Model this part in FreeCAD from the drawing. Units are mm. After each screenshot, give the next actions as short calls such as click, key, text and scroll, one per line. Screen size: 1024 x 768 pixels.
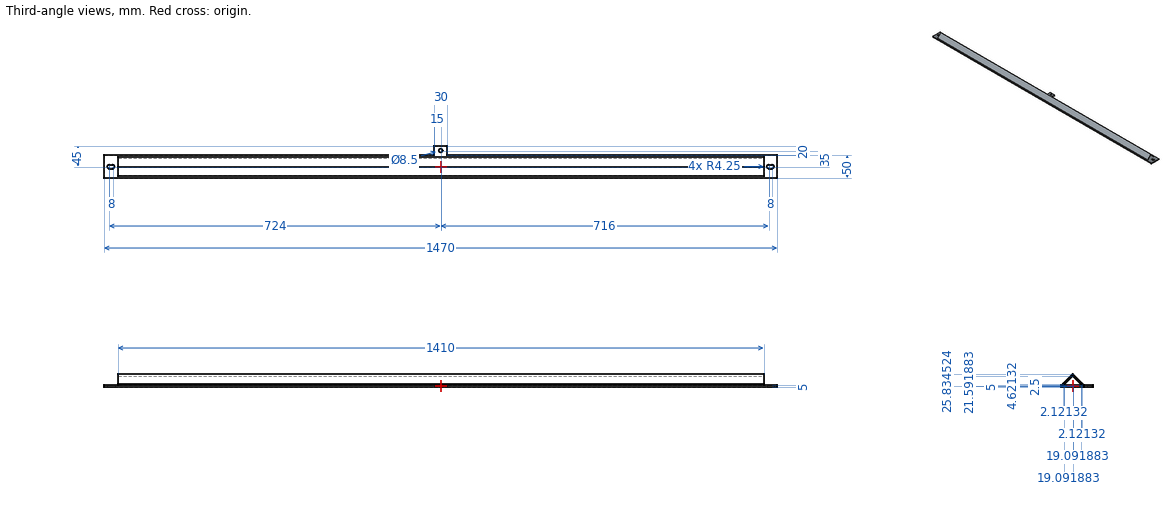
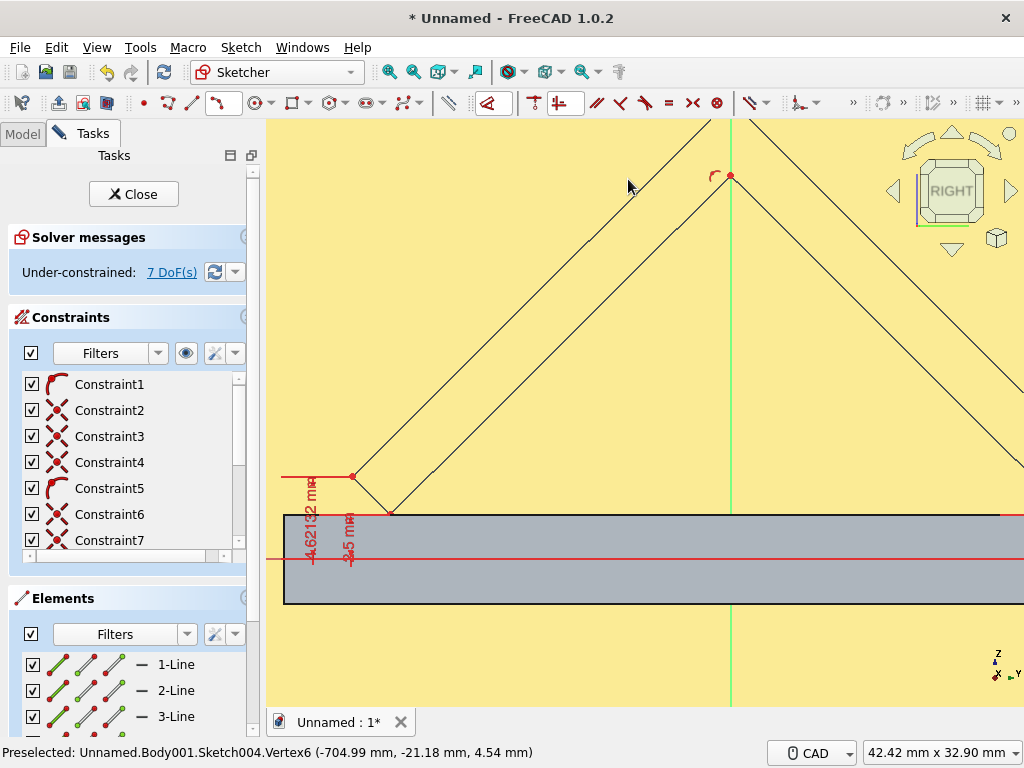
scroll(389, 516, down, 3)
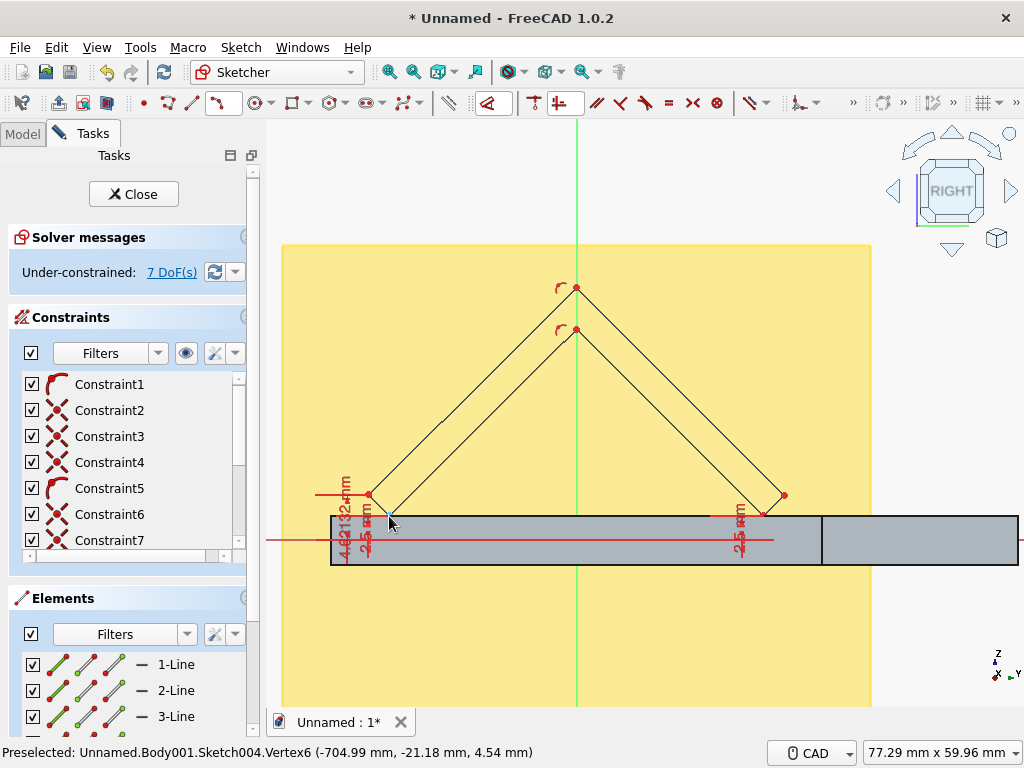
click(784, 496)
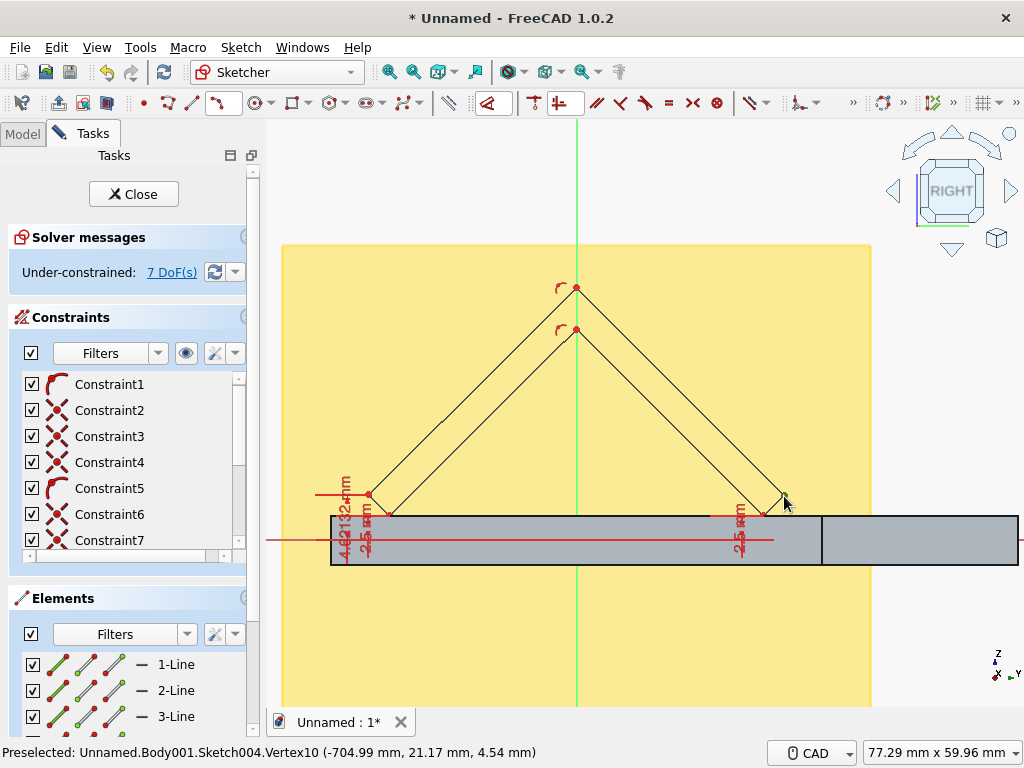
key(i)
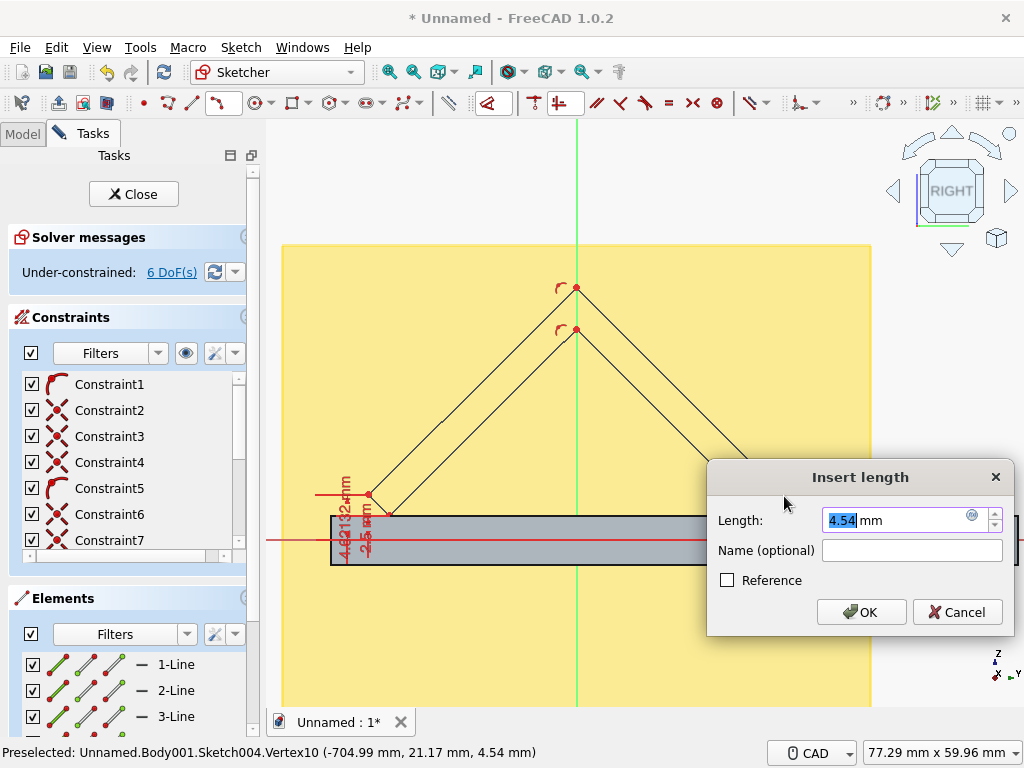
text(4.62132)
key(Return)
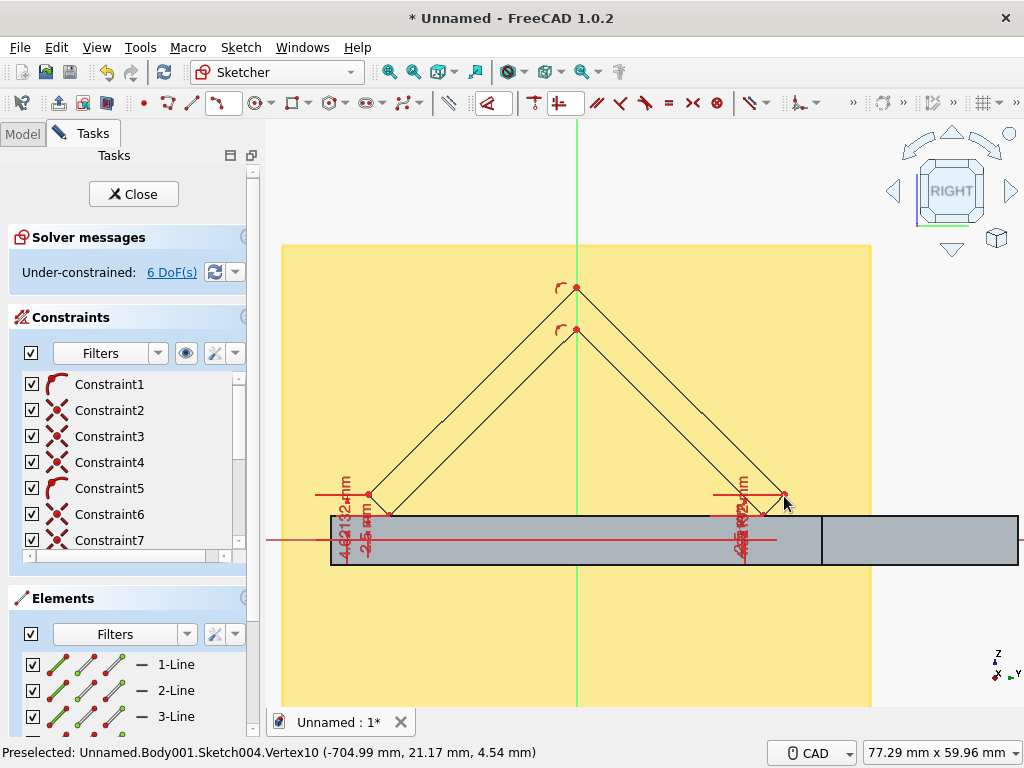
scroll(381, 507, up, 4)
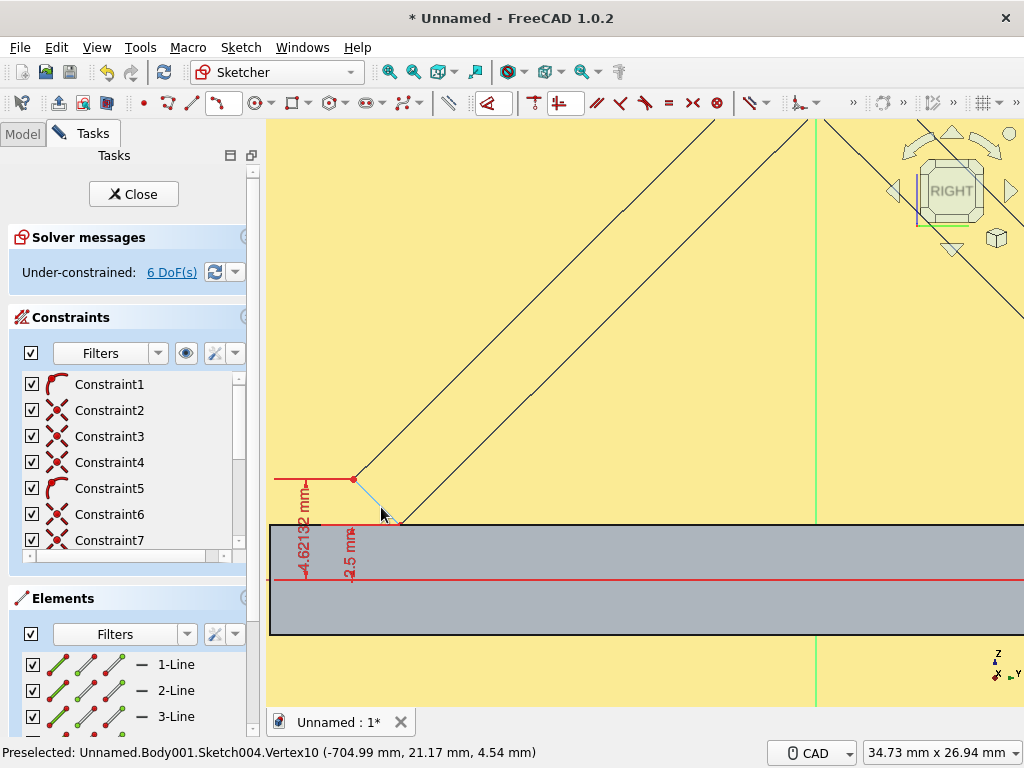
click(382, 507)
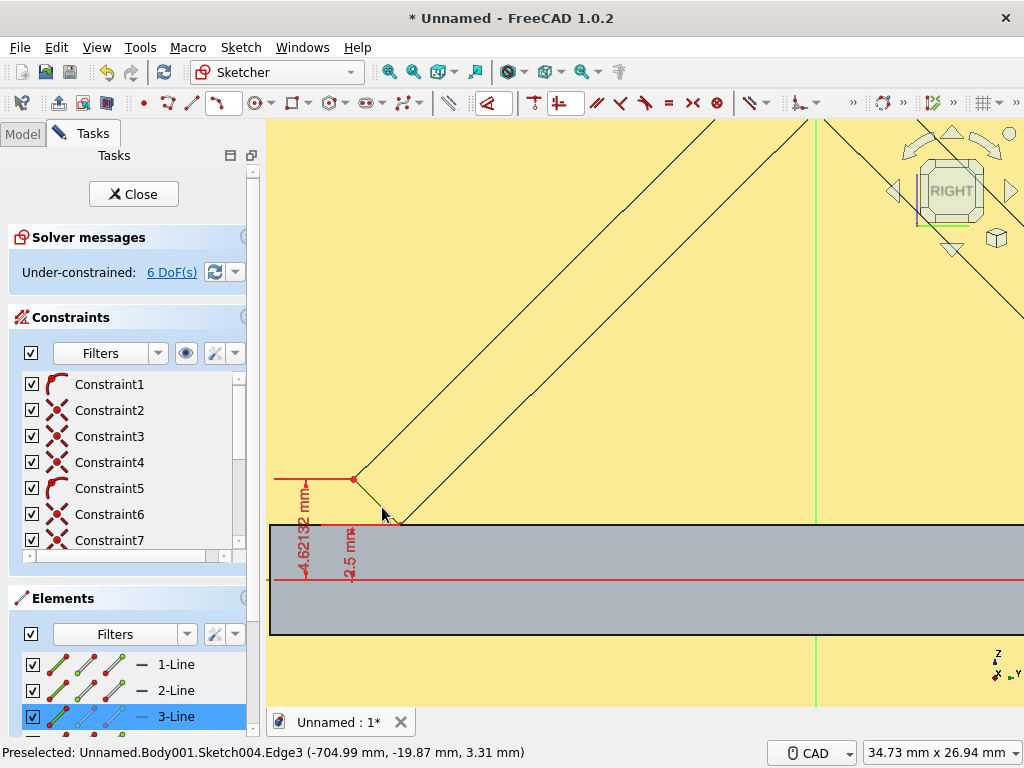
key(l)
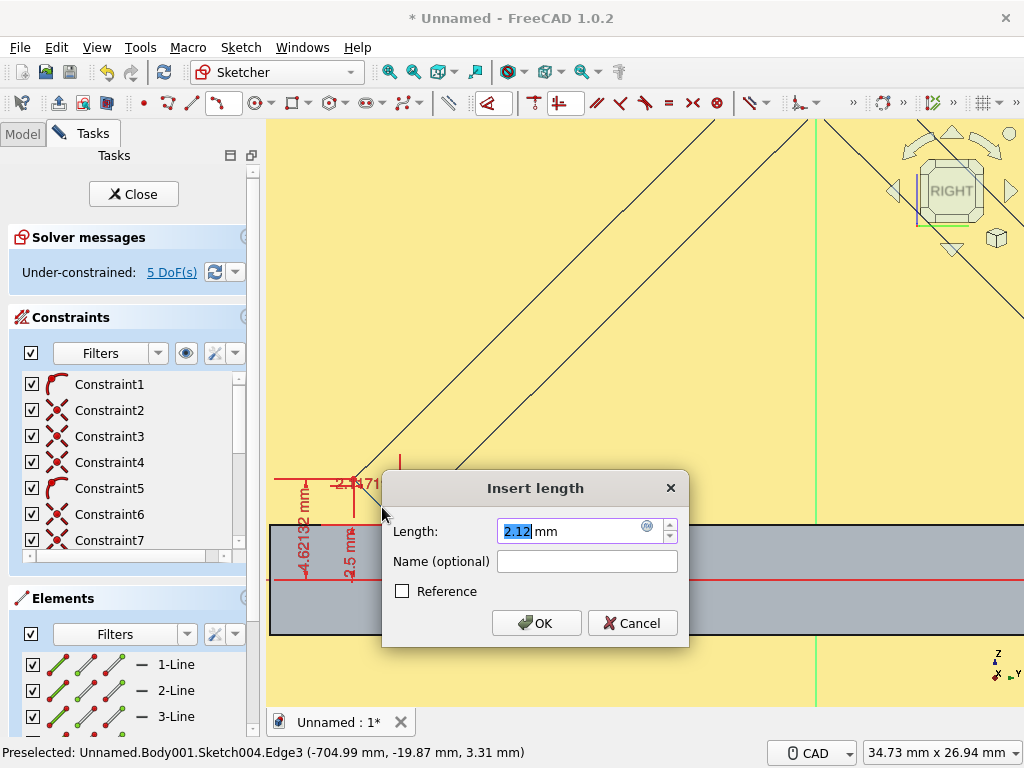
text(2.12132)
key(Return)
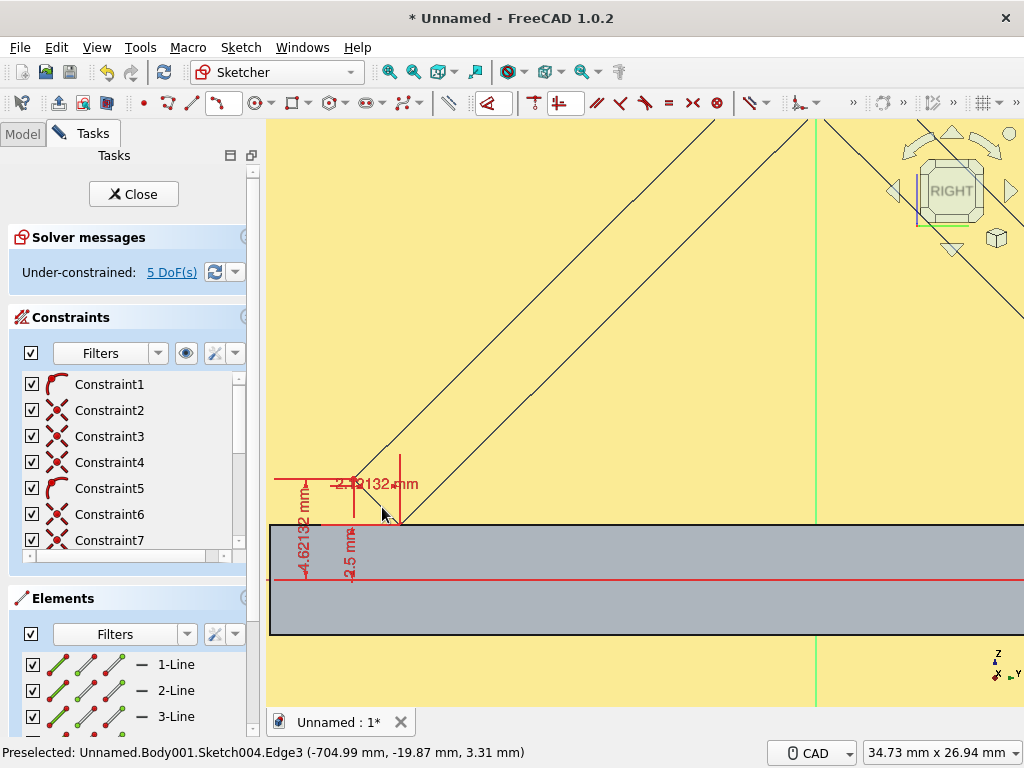
scroll(381, 507, down, 4)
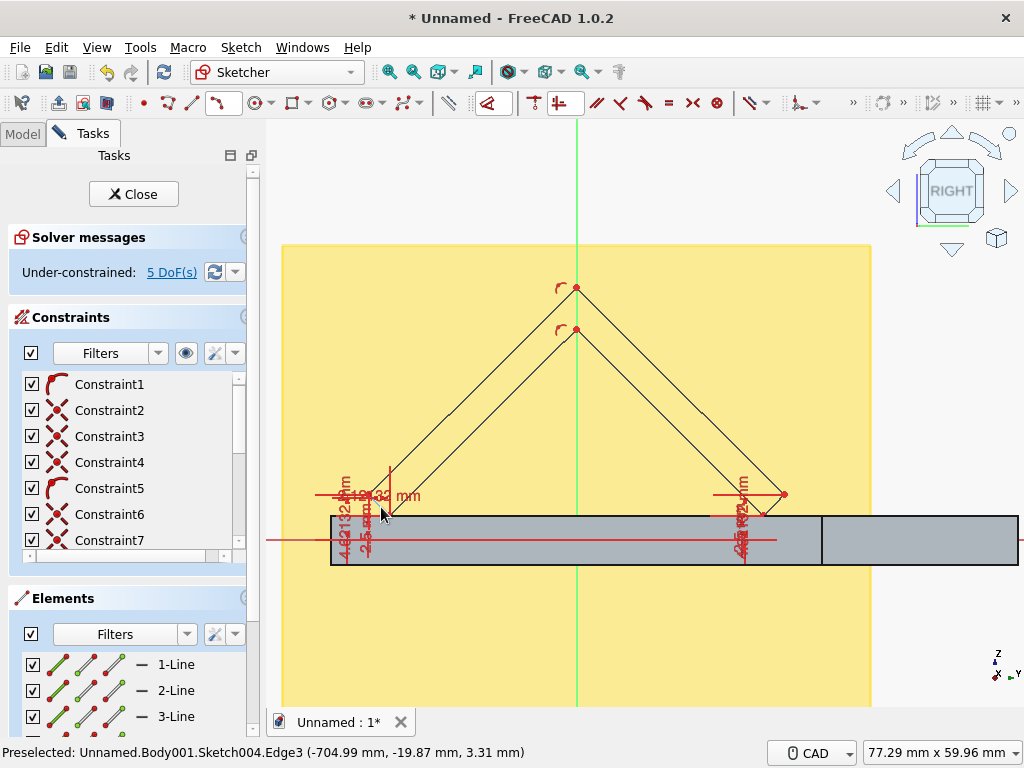
scroll(778, 501, up, 4)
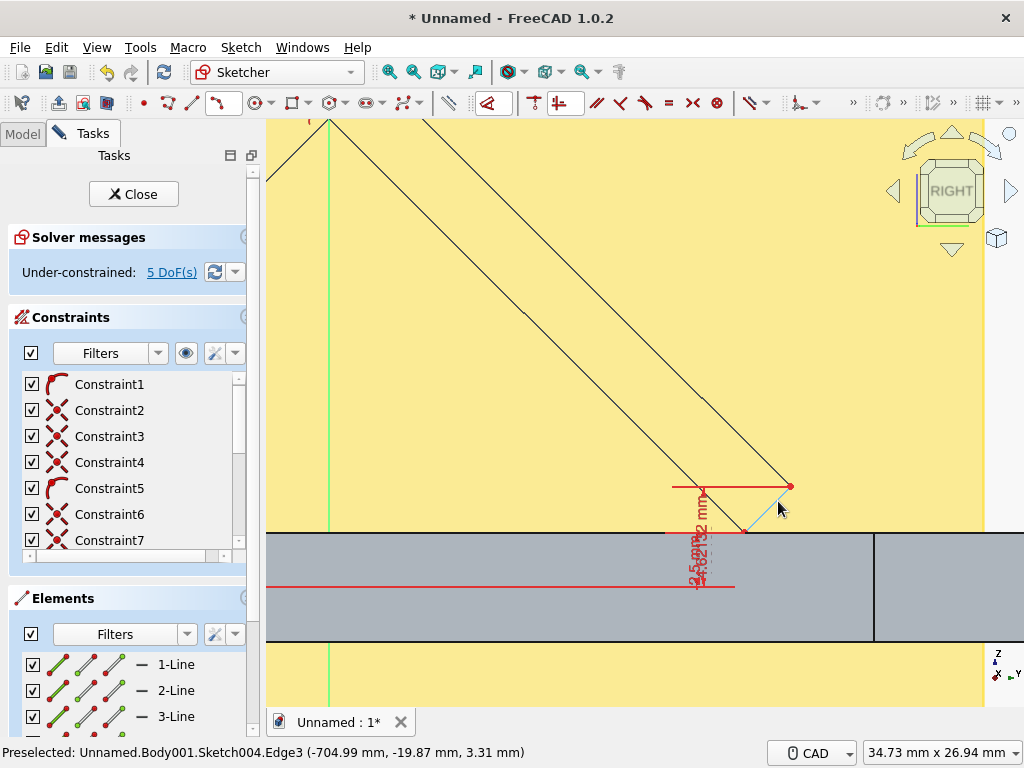
click(777, 500)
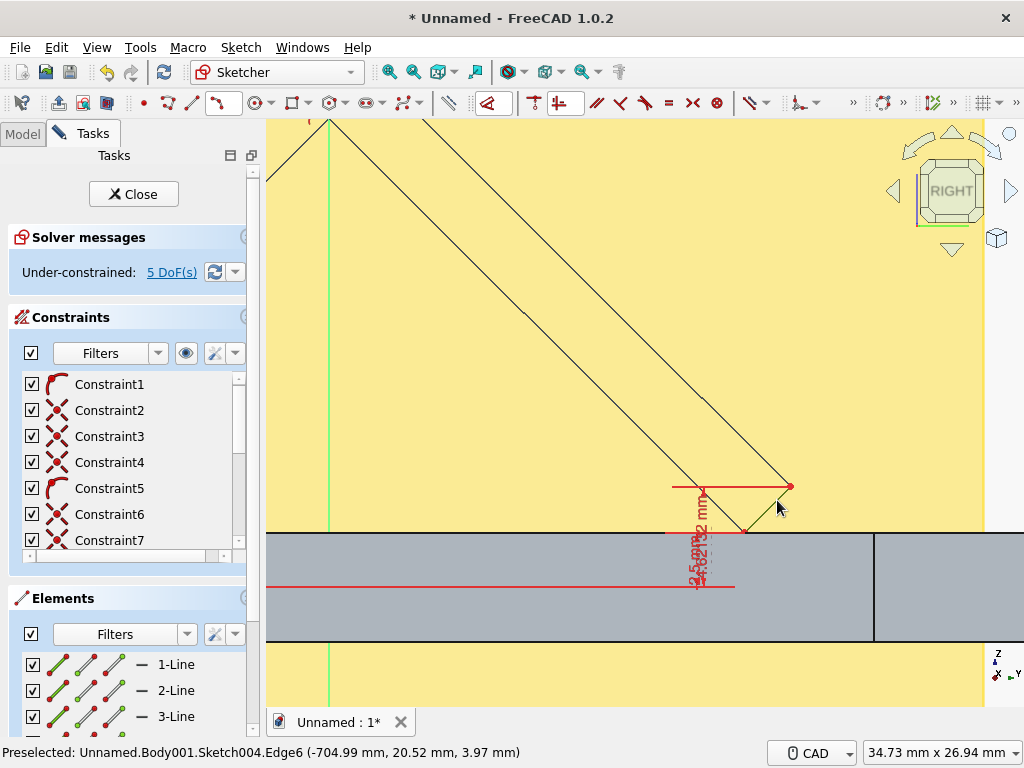
key(l)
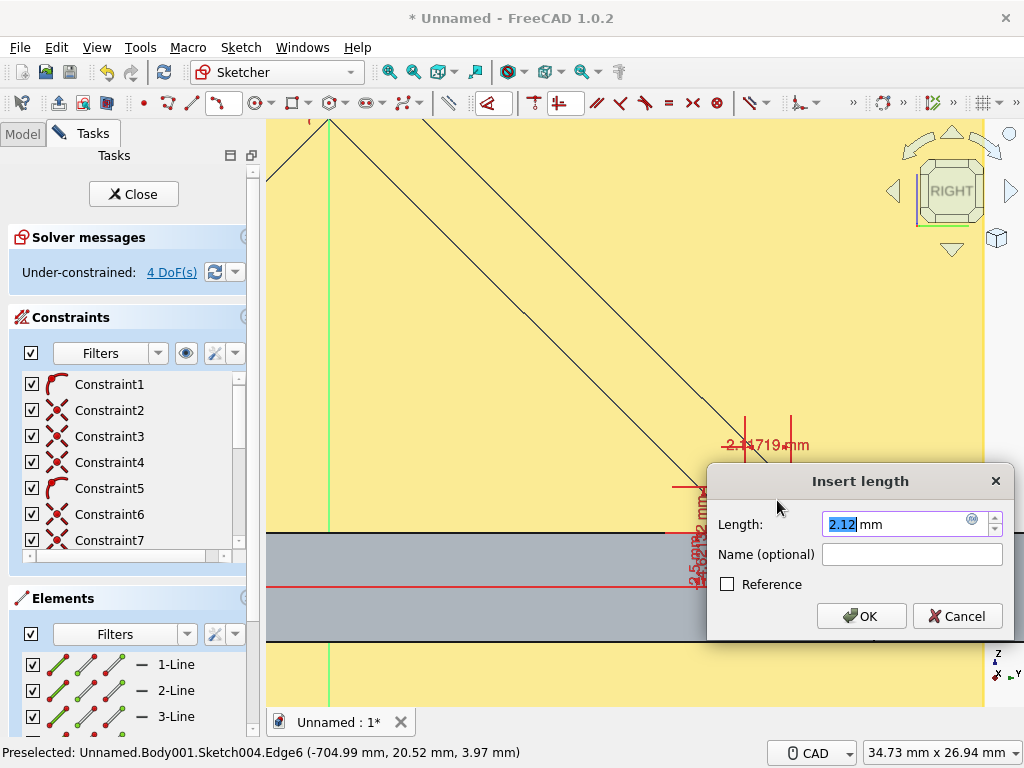
text(2.12132)
key(Return)